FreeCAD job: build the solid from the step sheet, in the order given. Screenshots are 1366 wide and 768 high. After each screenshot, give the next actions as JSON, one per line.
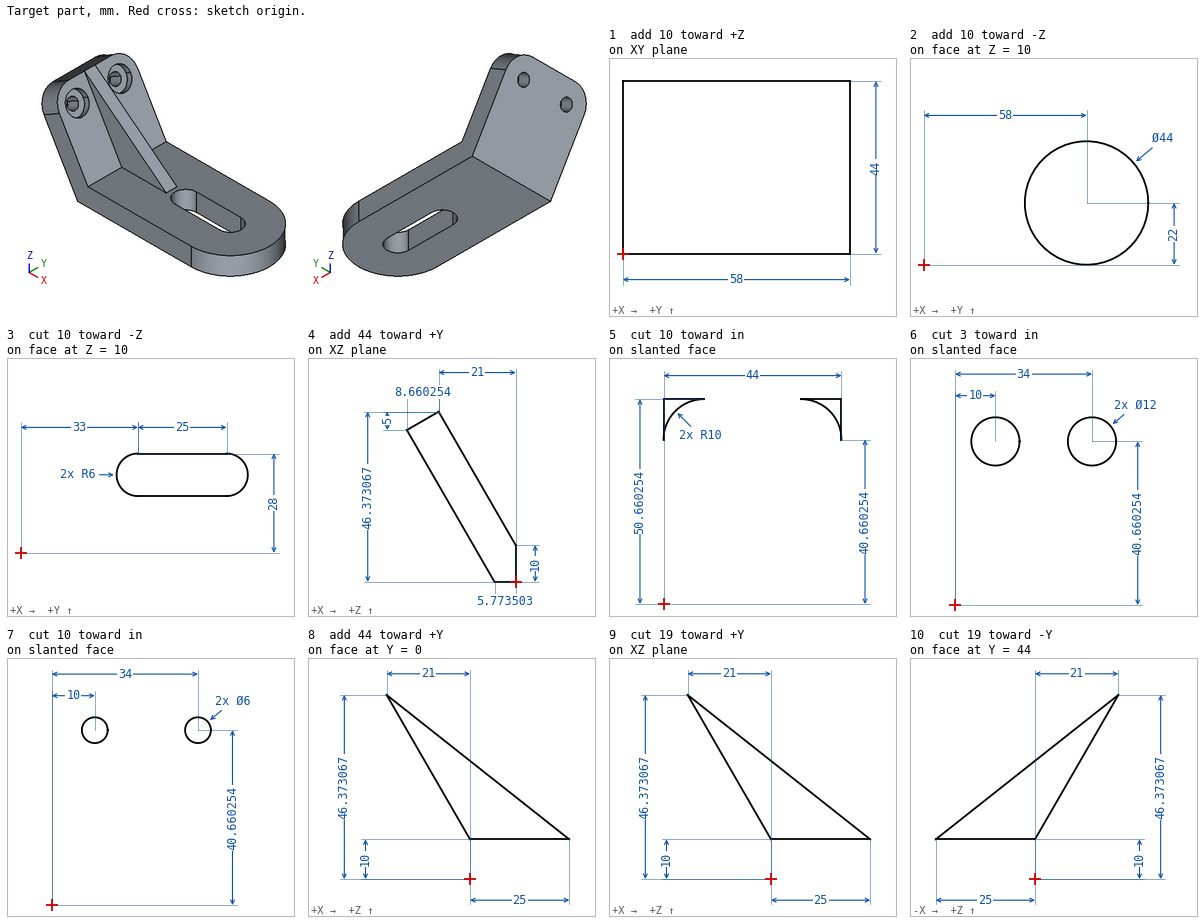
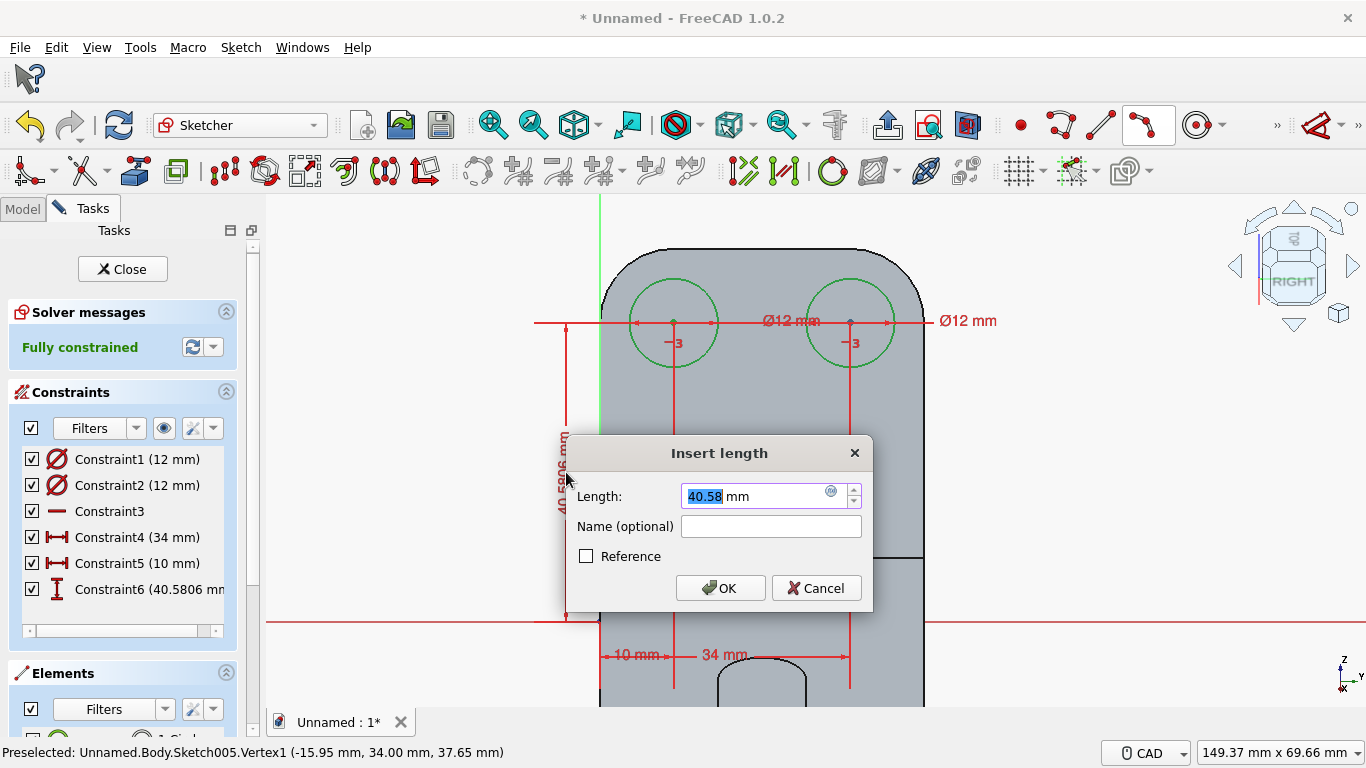
{"action": "type", "text": "40.660254"}
{"action": "key", "text": "Return"}
{"action": "key", "text": "Escape"}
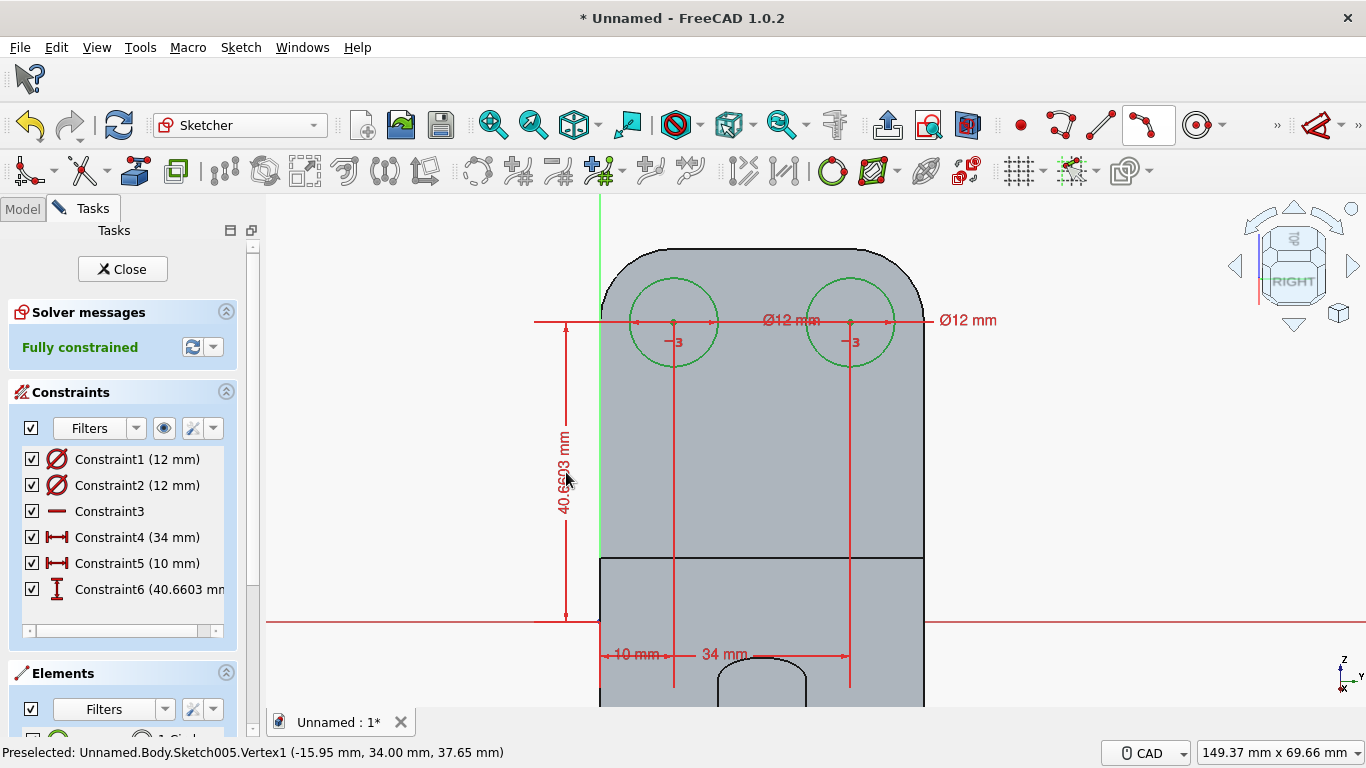
{"action": "left_click", "coordinate": [123, 269]}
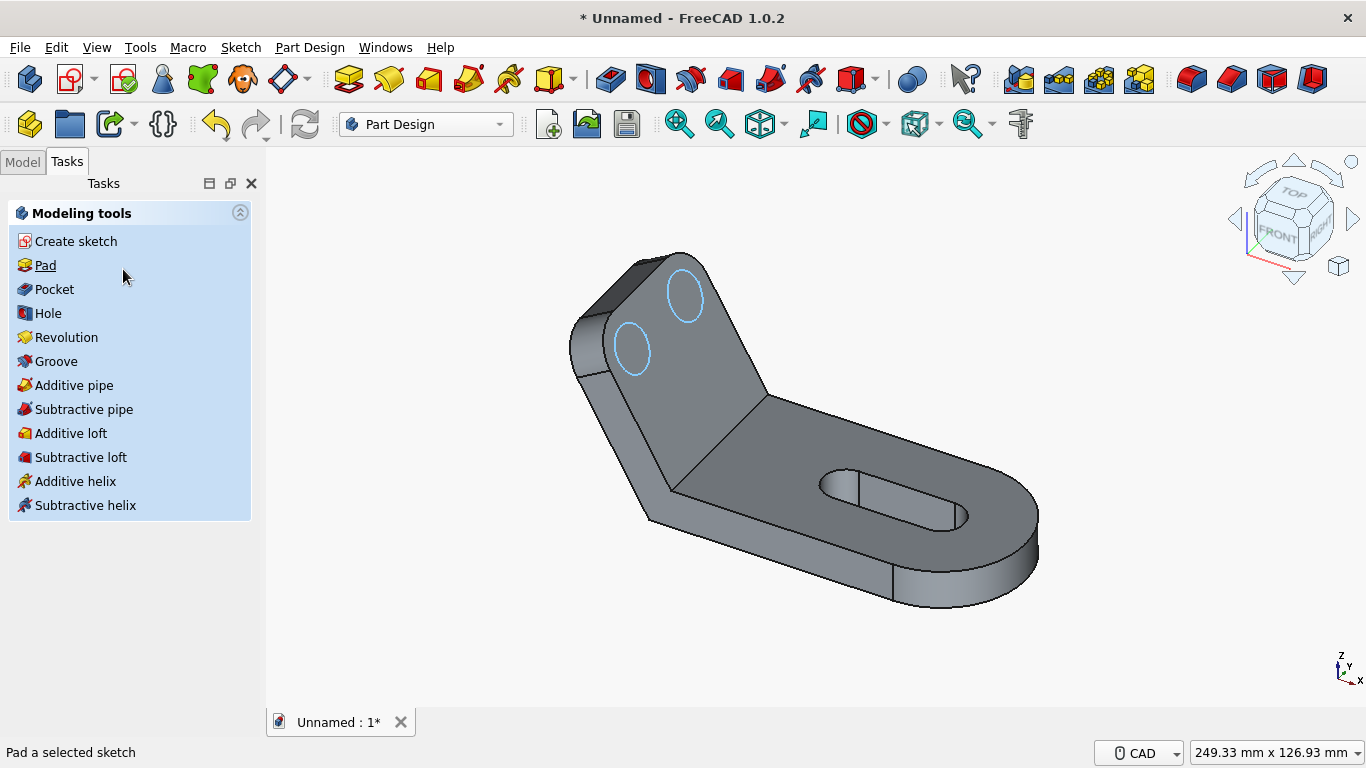
{"action": "left_click", "coordinate": [612, 80]}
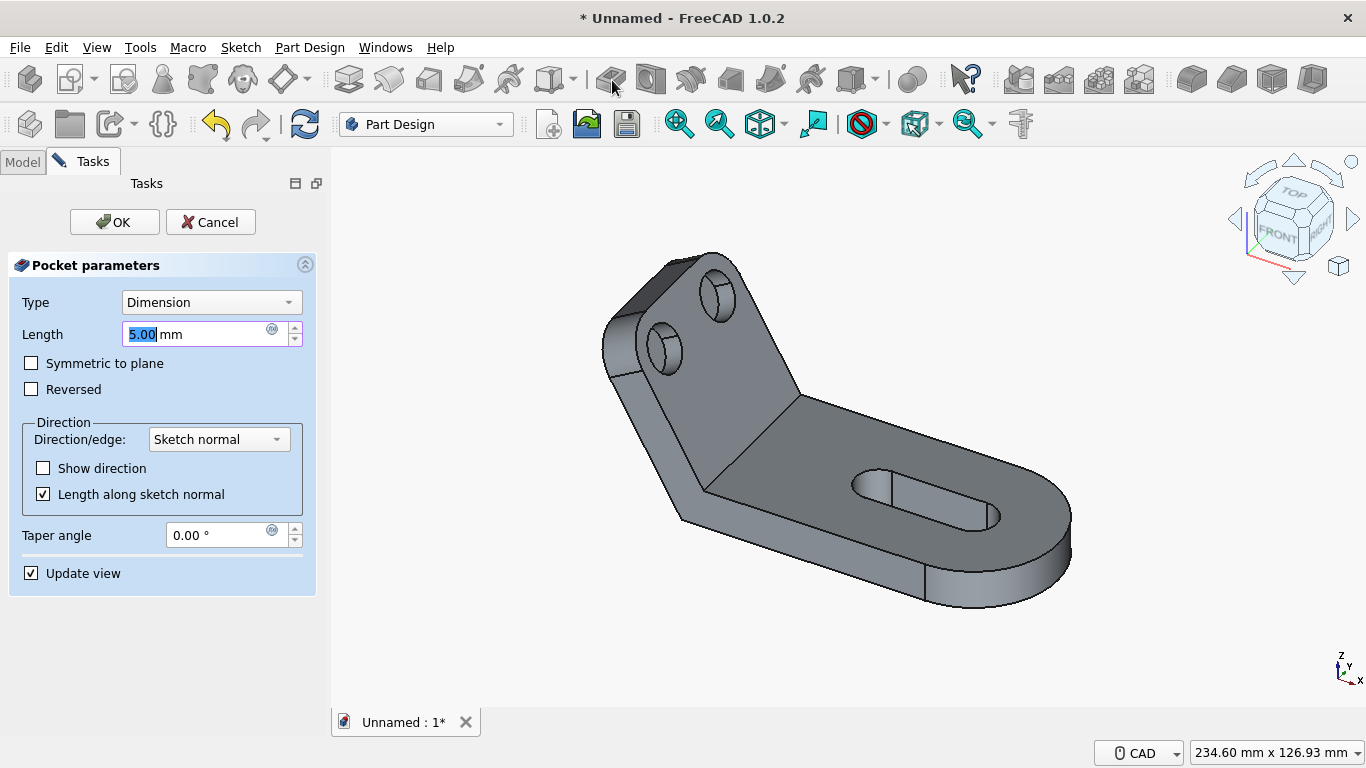
{"action": "type", "text": "3"}
{"action": "key", "text": "Tab"}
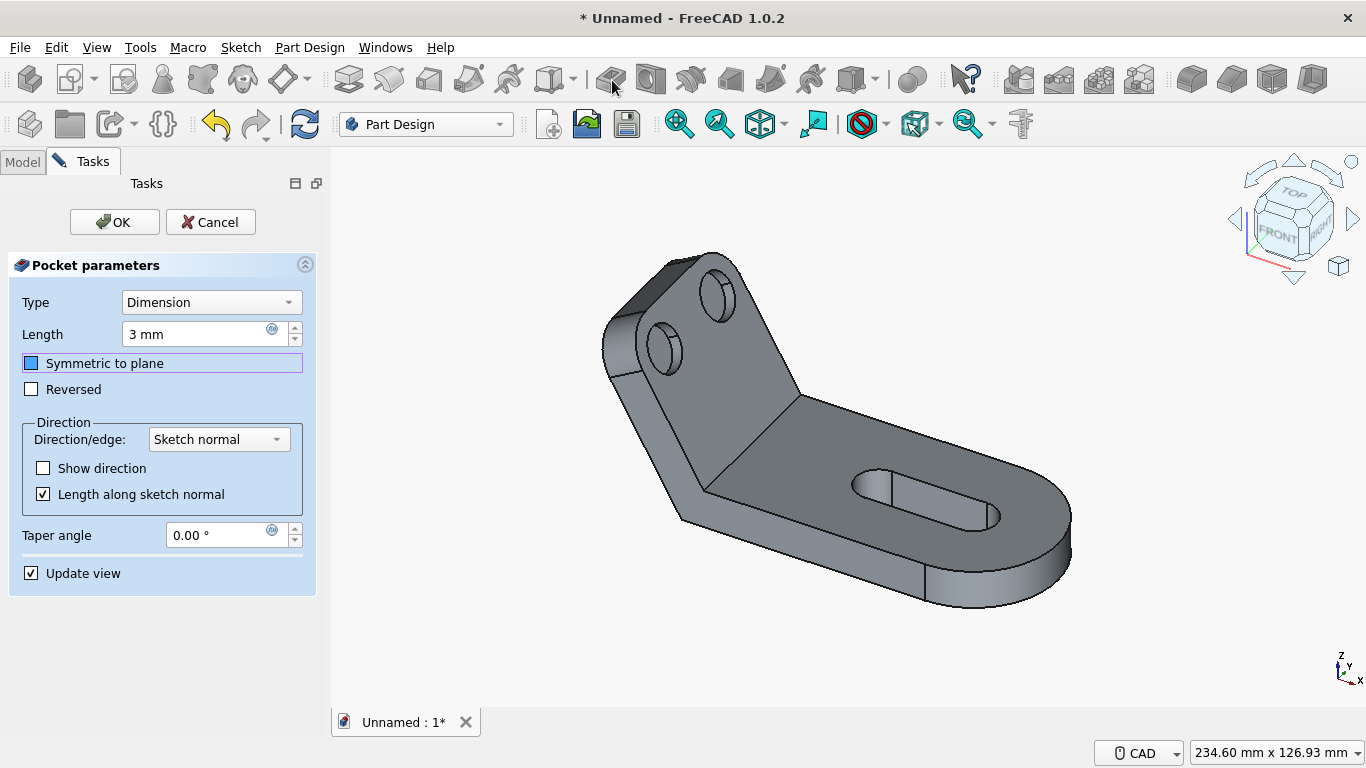
{"action": "left_click", "coordinate": [115, 222]}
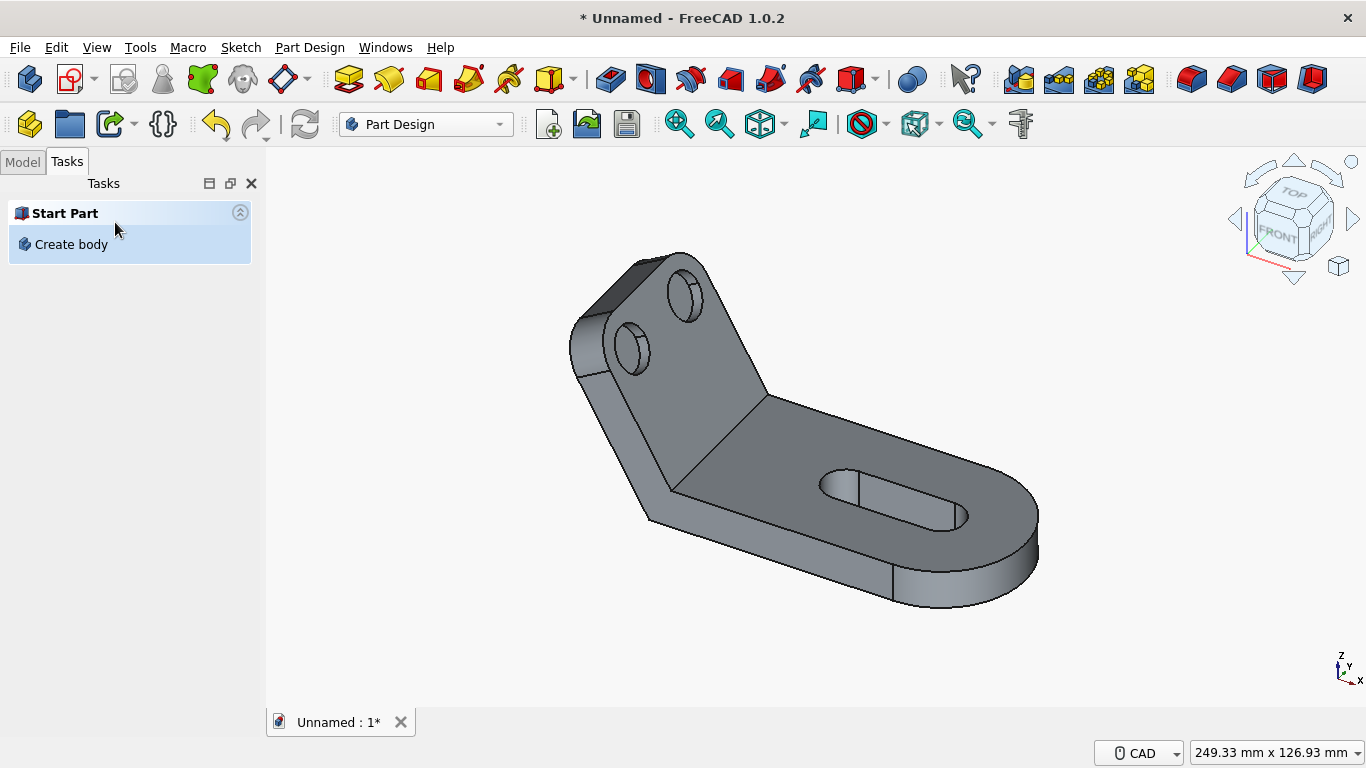
{"action": "left_click", "coordinate": [626, 346]}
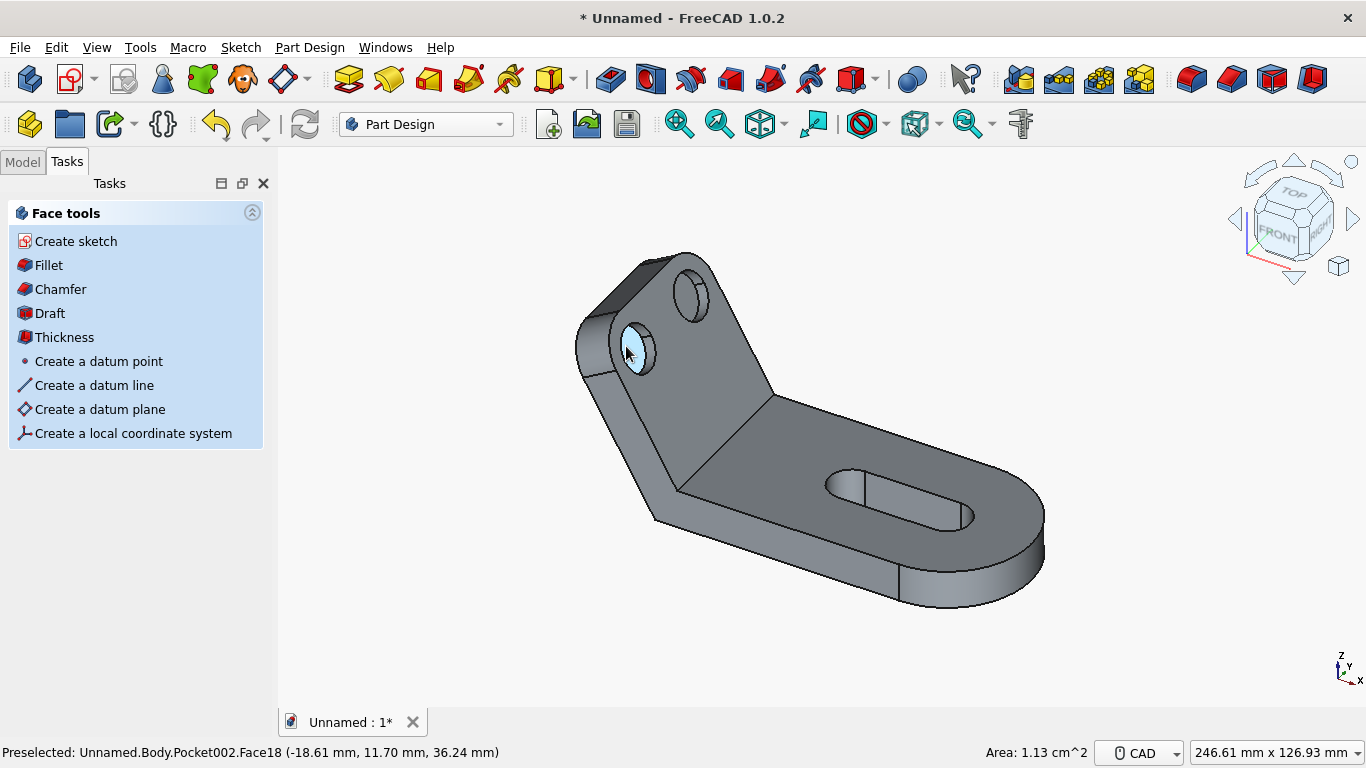
{"action": "left_click", "coordinate": [70, 80]}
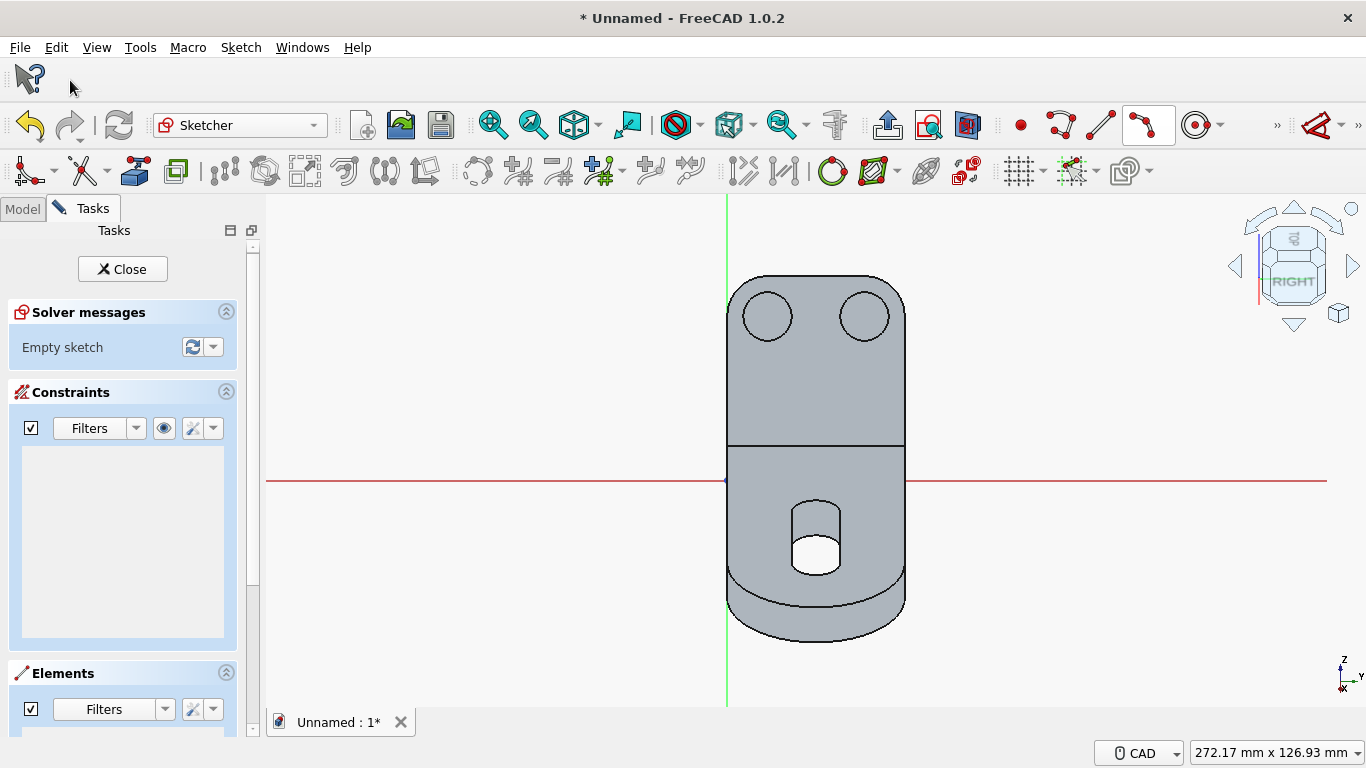
{"action": "scroll", "coordinate": [868, 322], "scroll_direction": "up", "scroll_amount": 3}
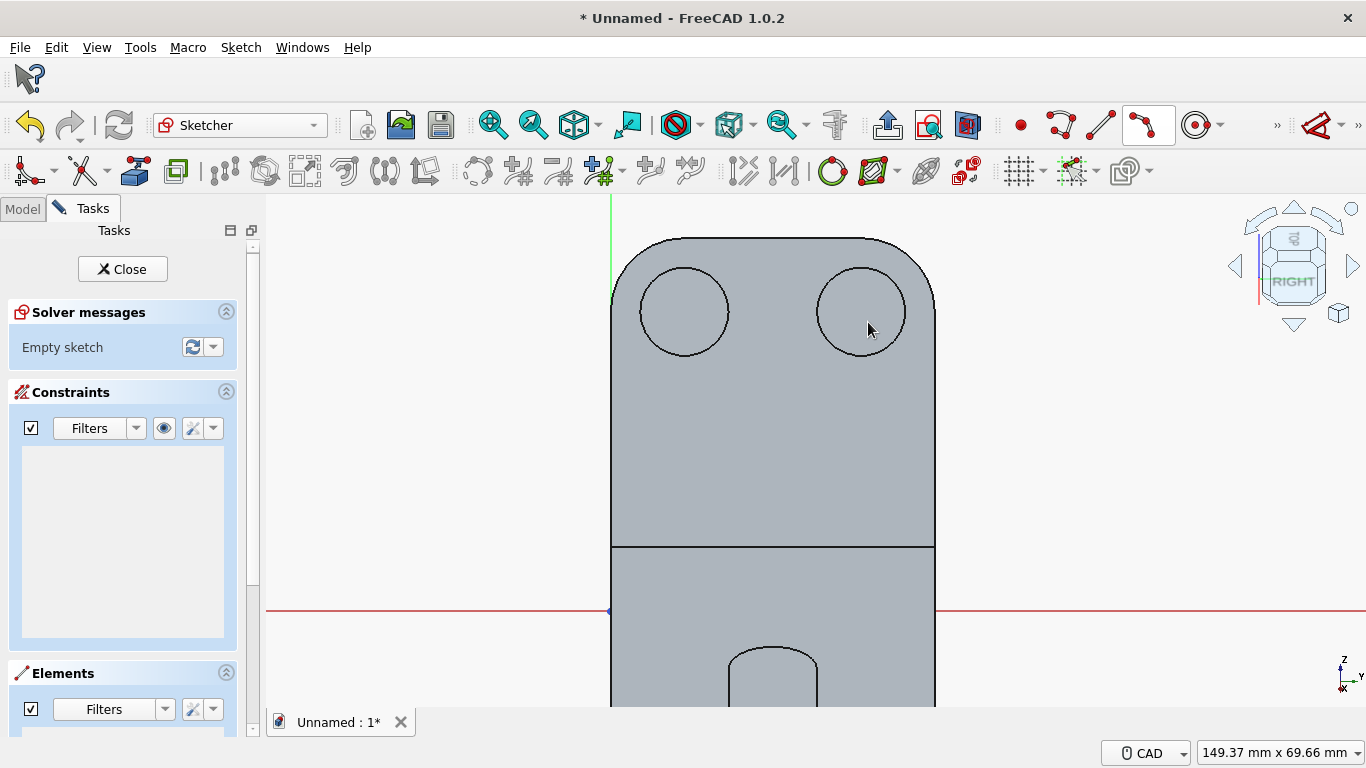
{"action": "key", "text": "g c"}